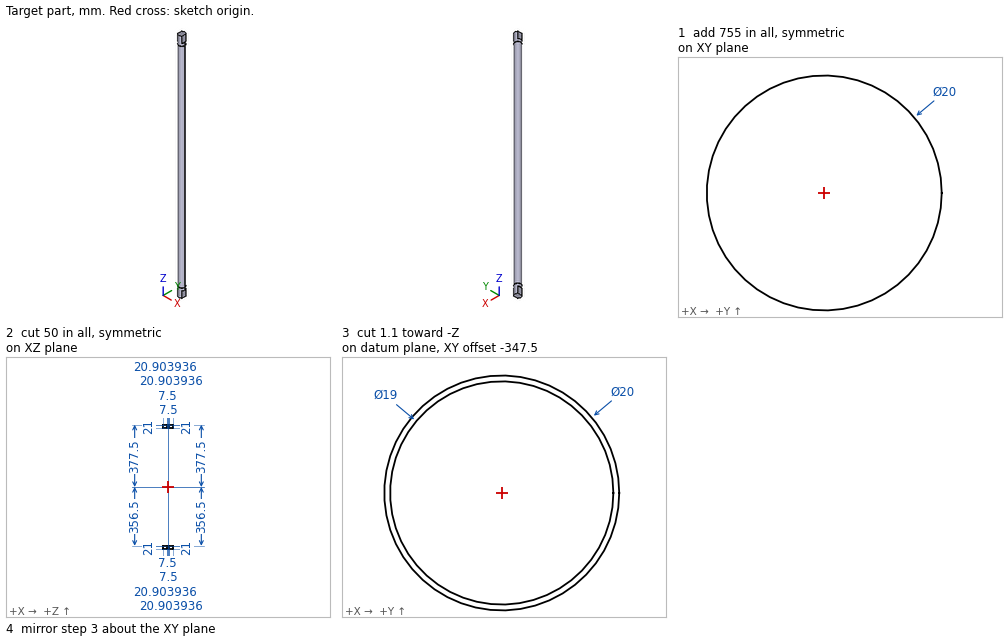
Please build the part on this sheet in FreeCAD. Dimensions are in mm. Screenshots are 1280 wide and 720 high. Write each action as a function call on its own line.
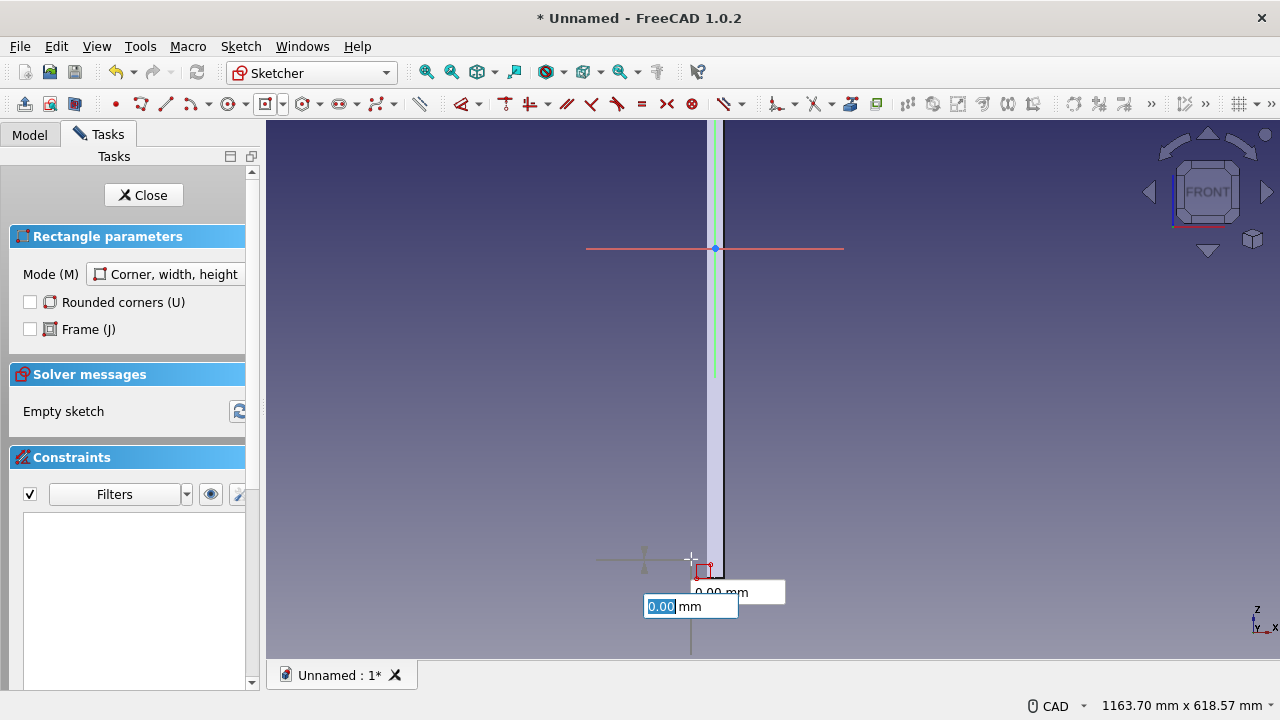
scroll(709, 578, up, 5)
move(708, 575)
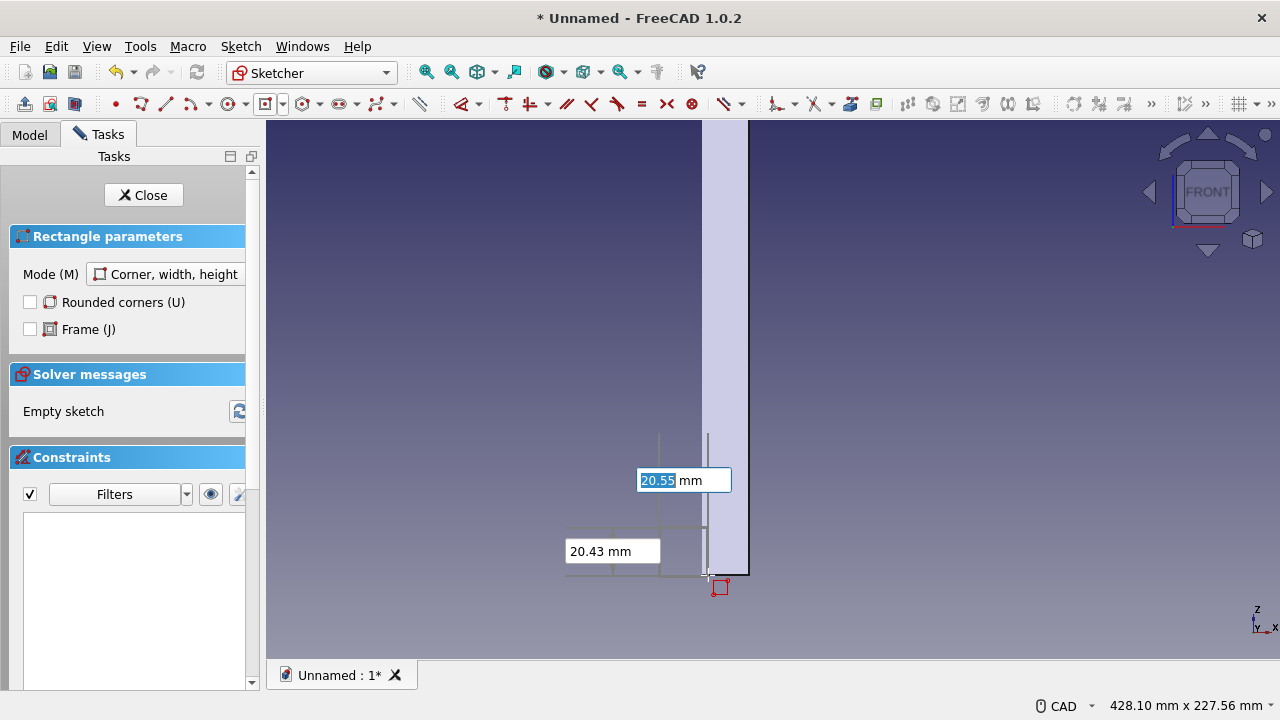
text(20.903936)
key(Tab)
text(21)
key(Return)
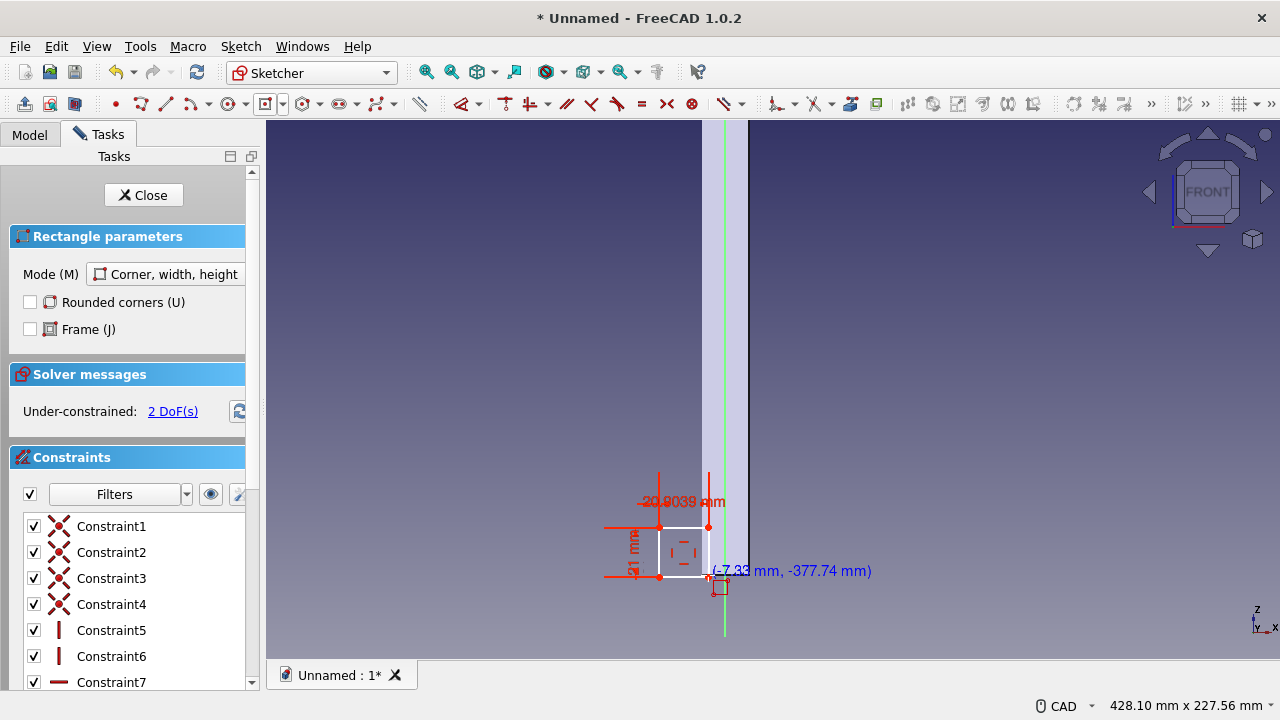
click(743, 526)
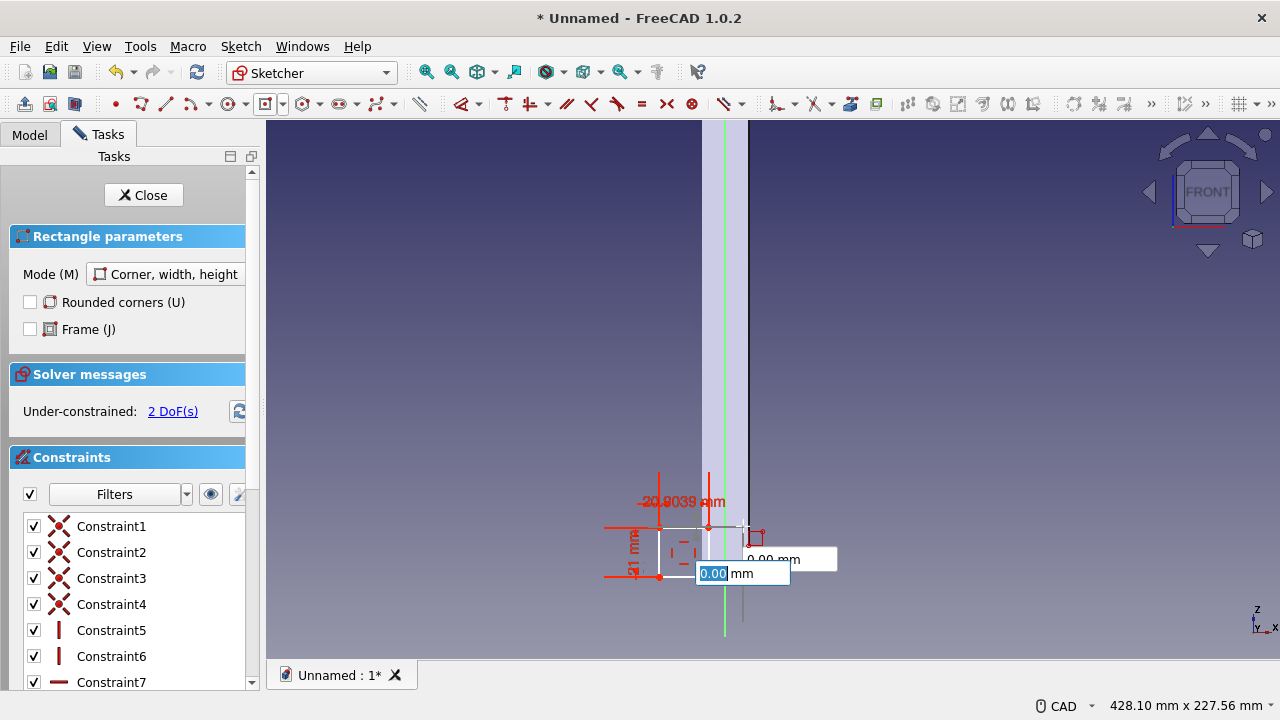
scroll(699, 569, down, 8)
move(718, 571)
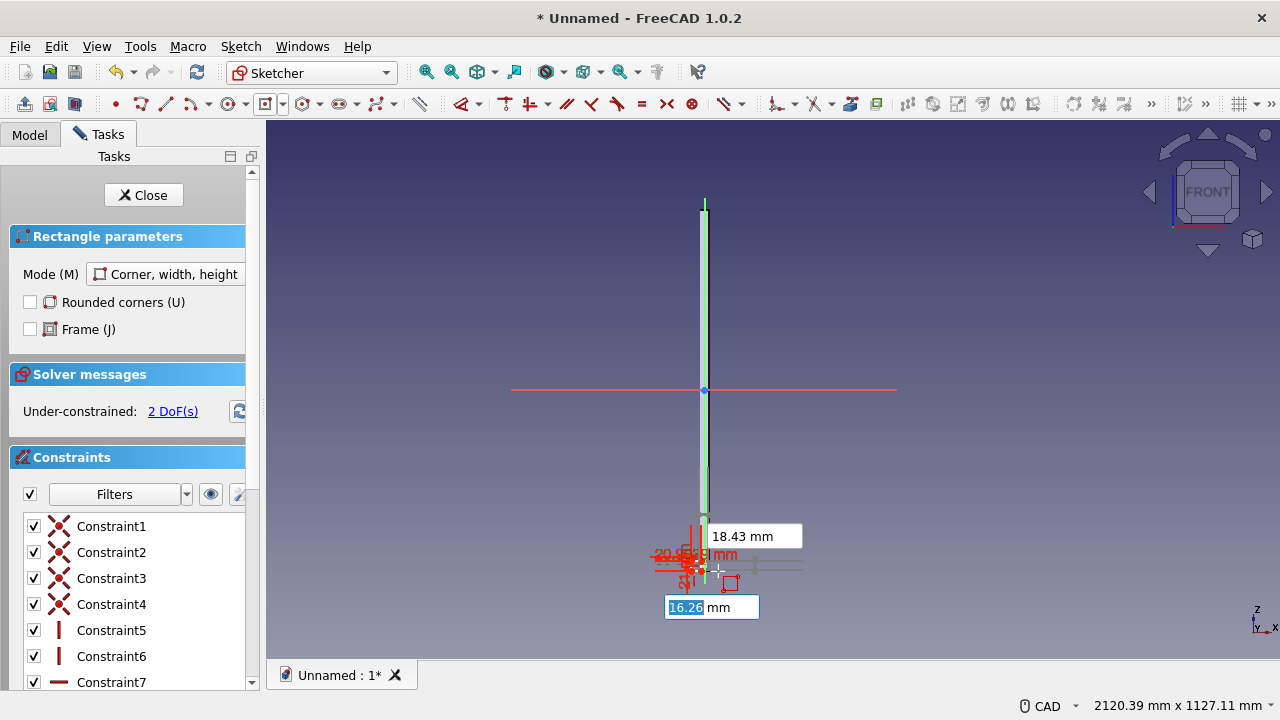
text(20.903936)
key(Tab)
text(21)
key(Return)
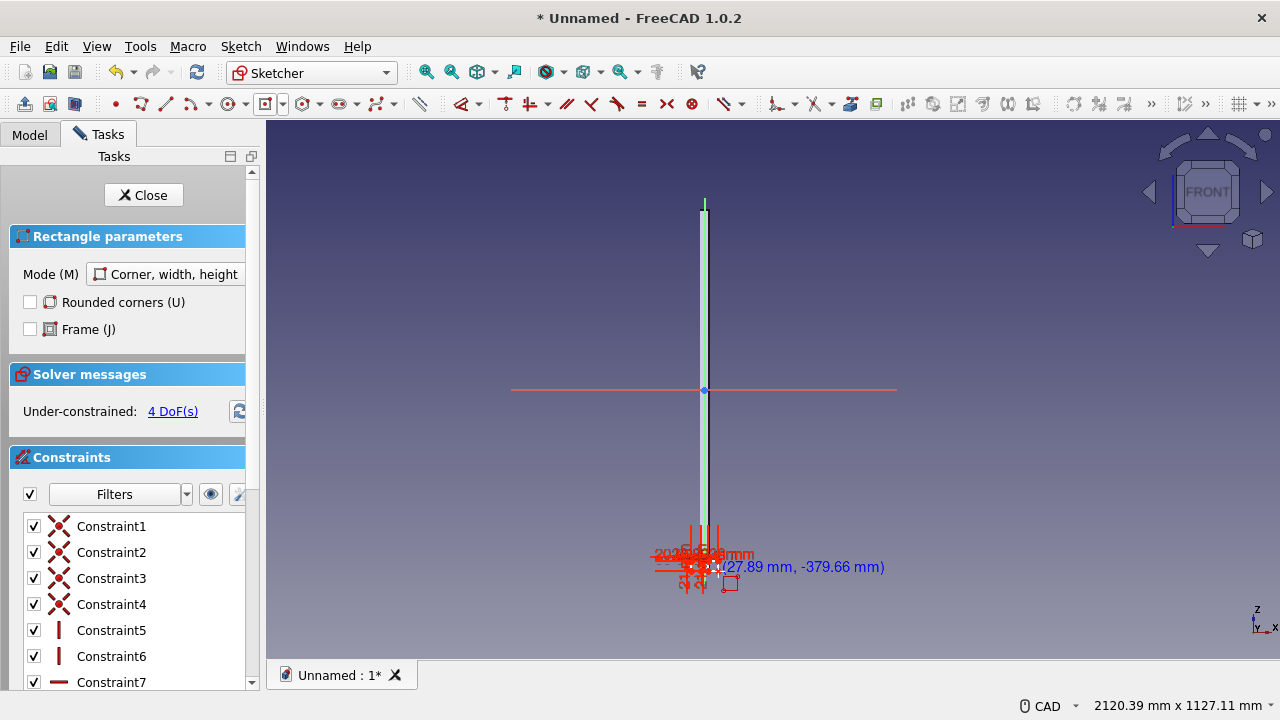
scroll(708, 210, up, 8)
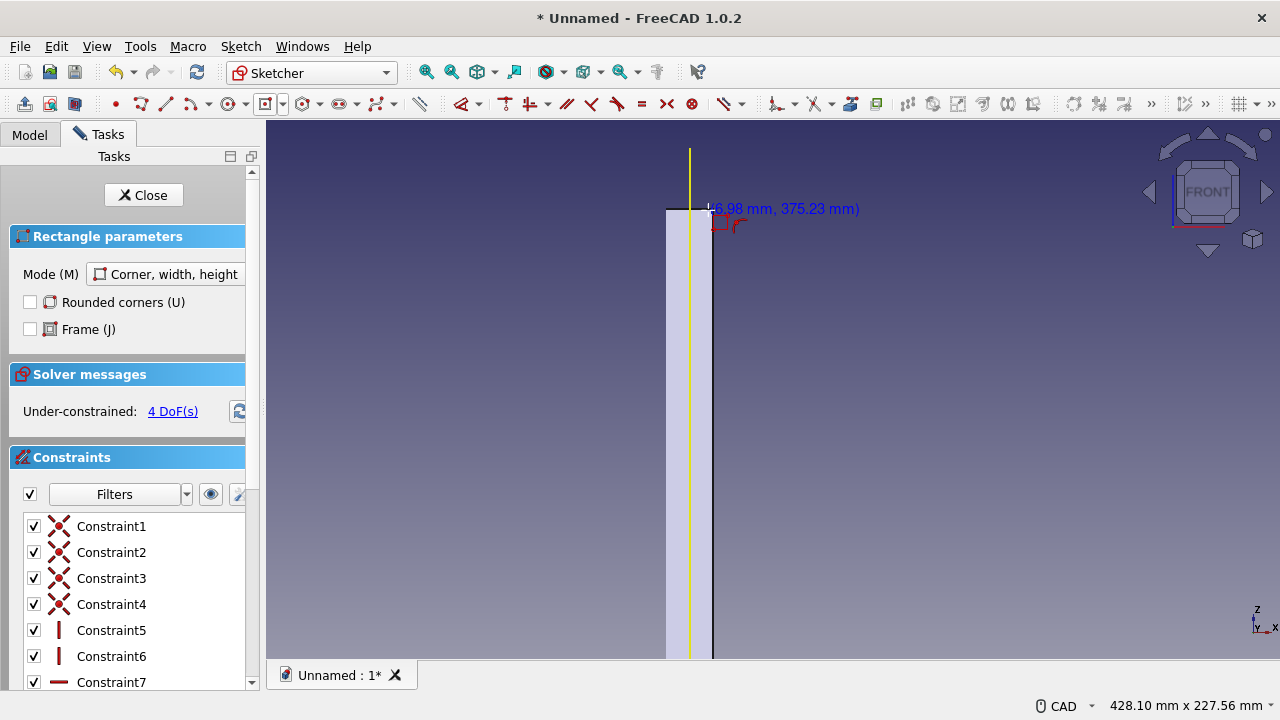
click(708, 209)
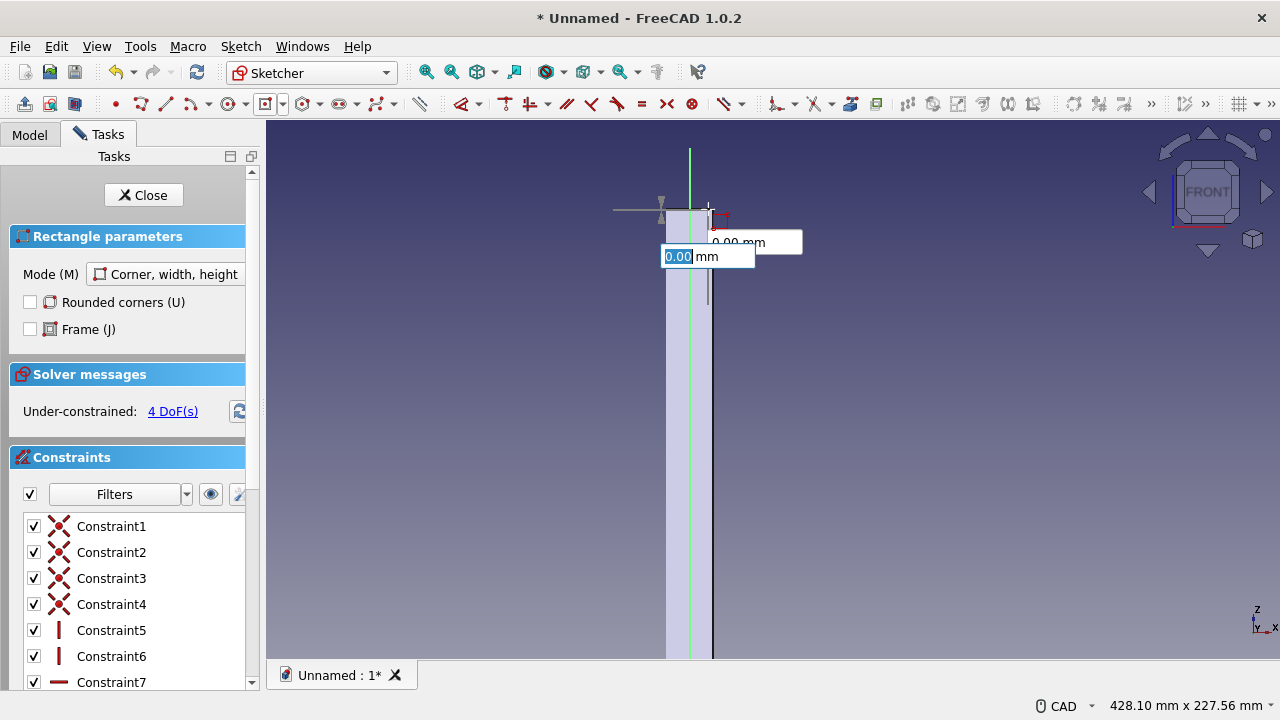
scroll(708, 209, down, 8)
move(718, 219)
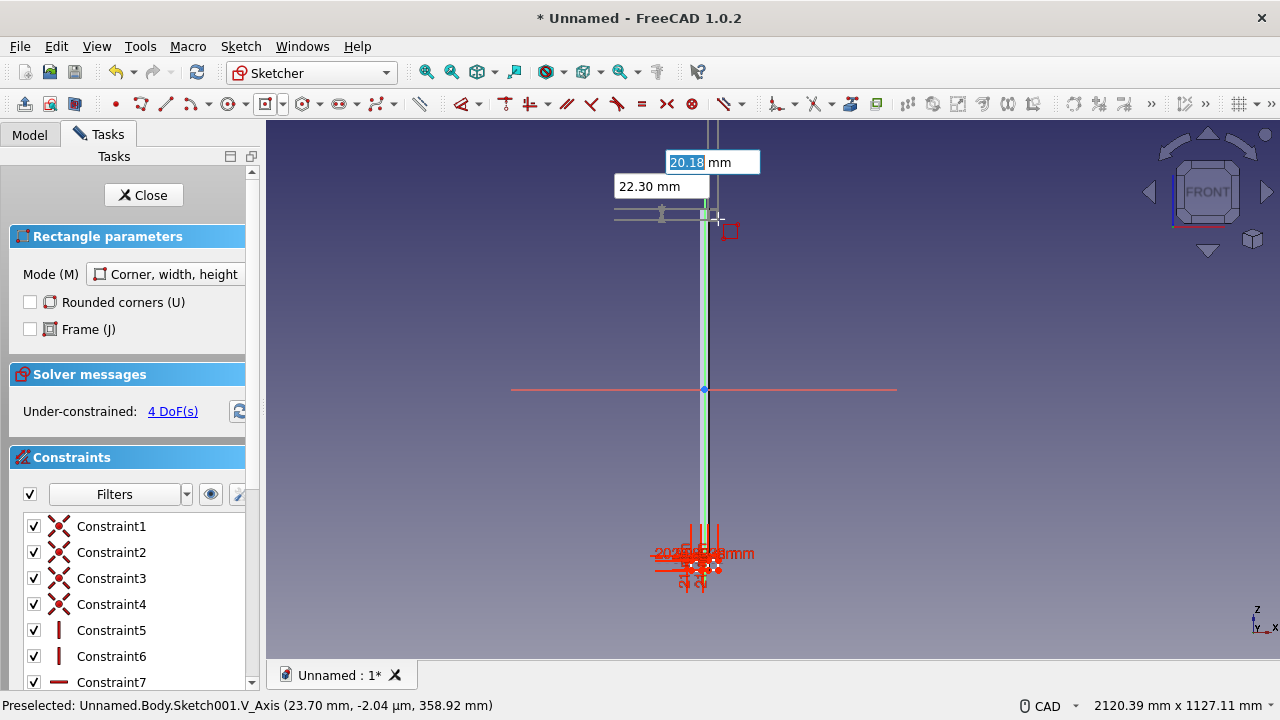
text(20.903936)
key(Tab)
text(21)
key(Return)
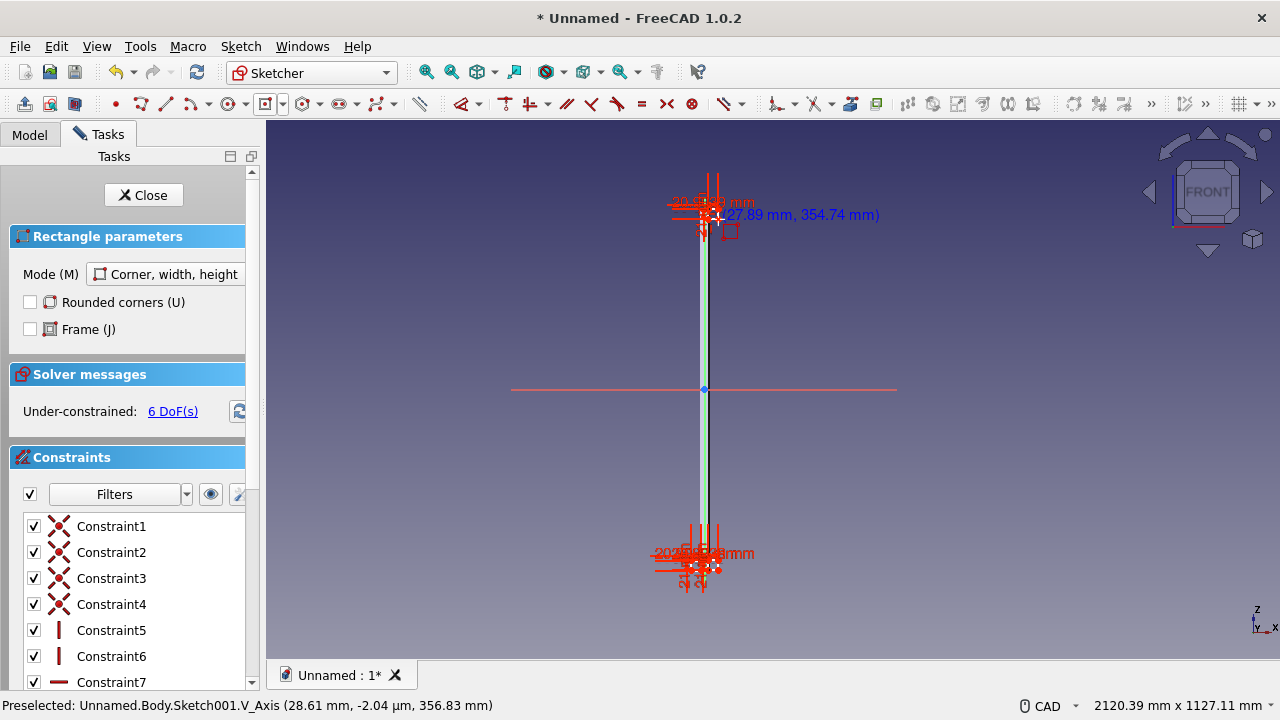
scroll(691, 209, up, 3)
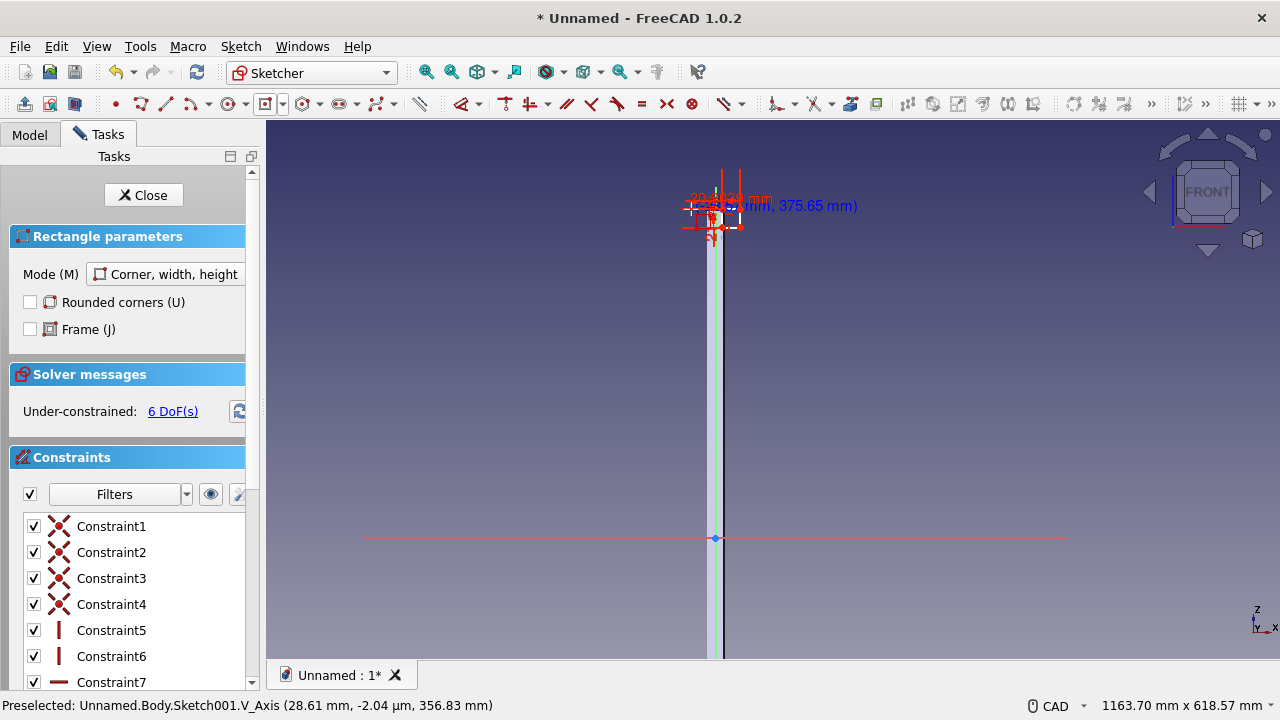
click(691, 209)